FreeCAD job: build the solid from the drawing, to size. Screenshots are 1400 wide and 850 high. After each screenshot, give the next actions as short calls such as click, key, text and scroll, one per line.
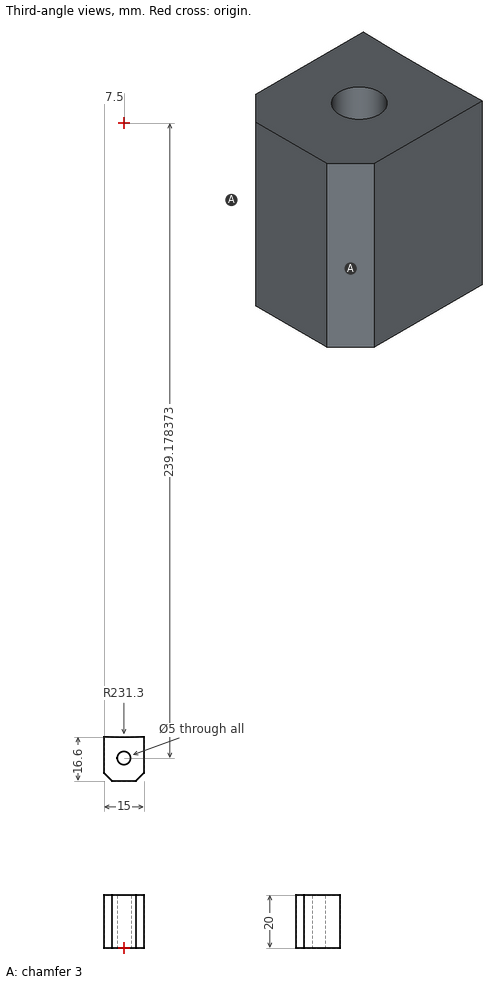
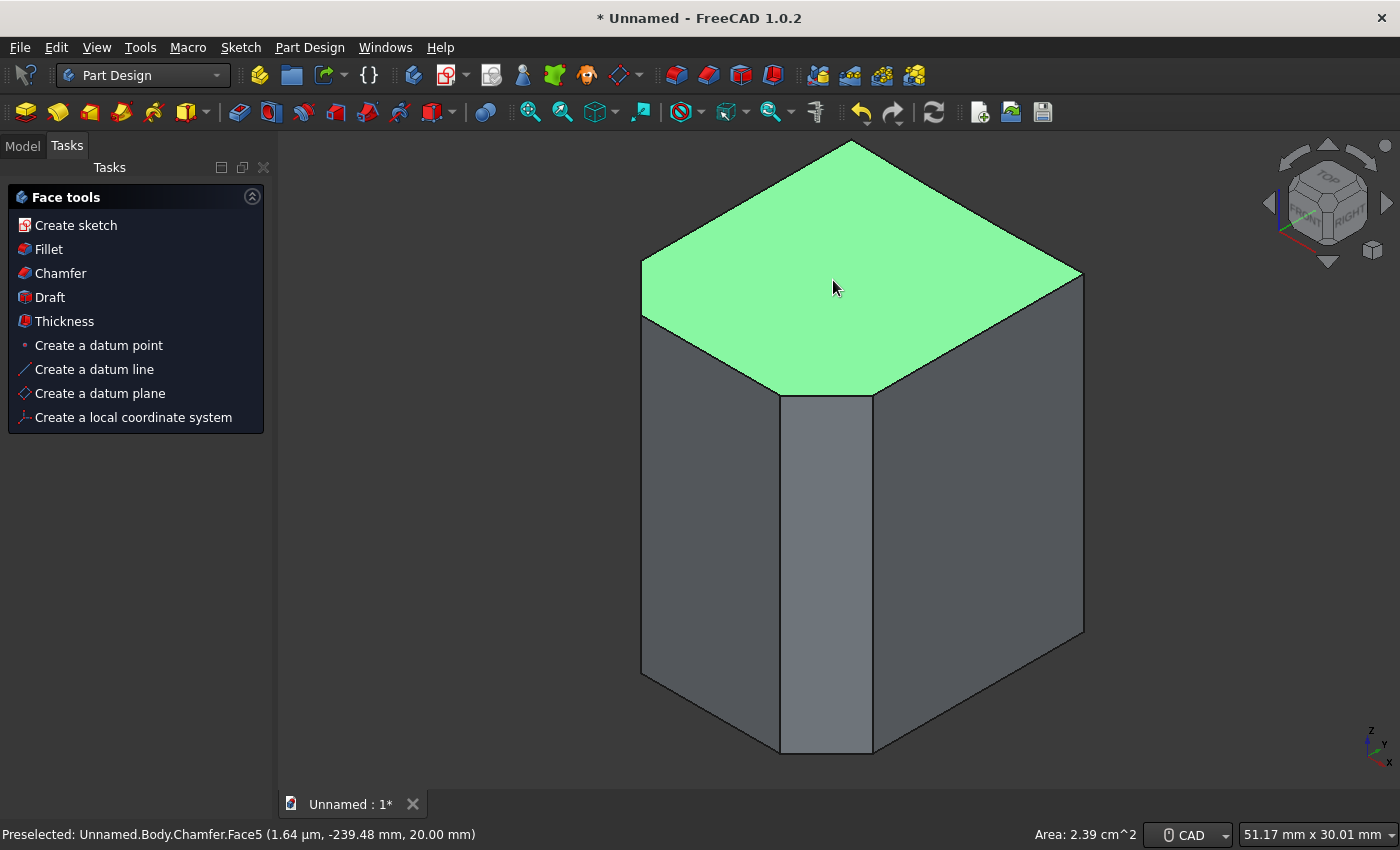
click(446, 76)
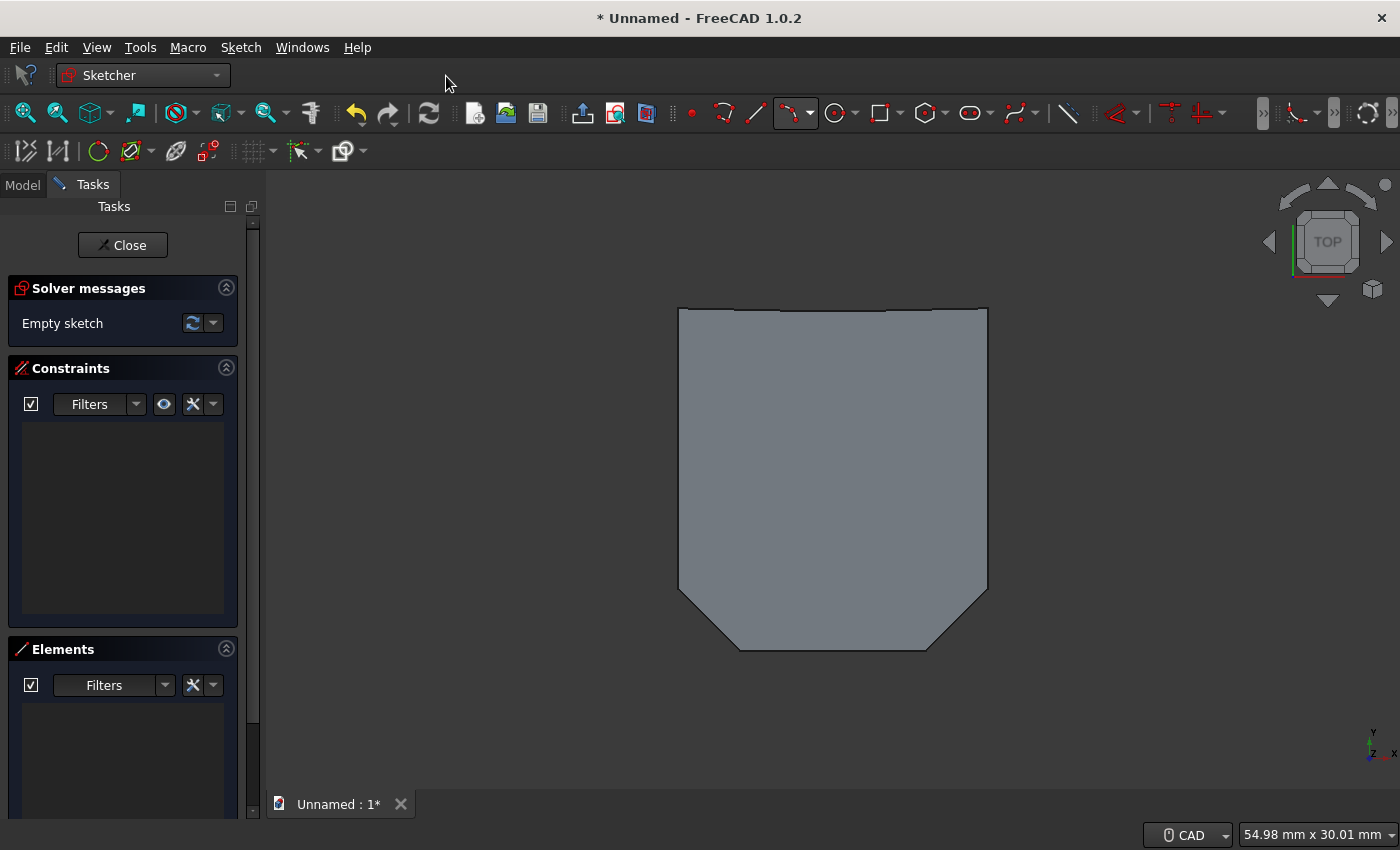
scroll(855, 471, up, 7)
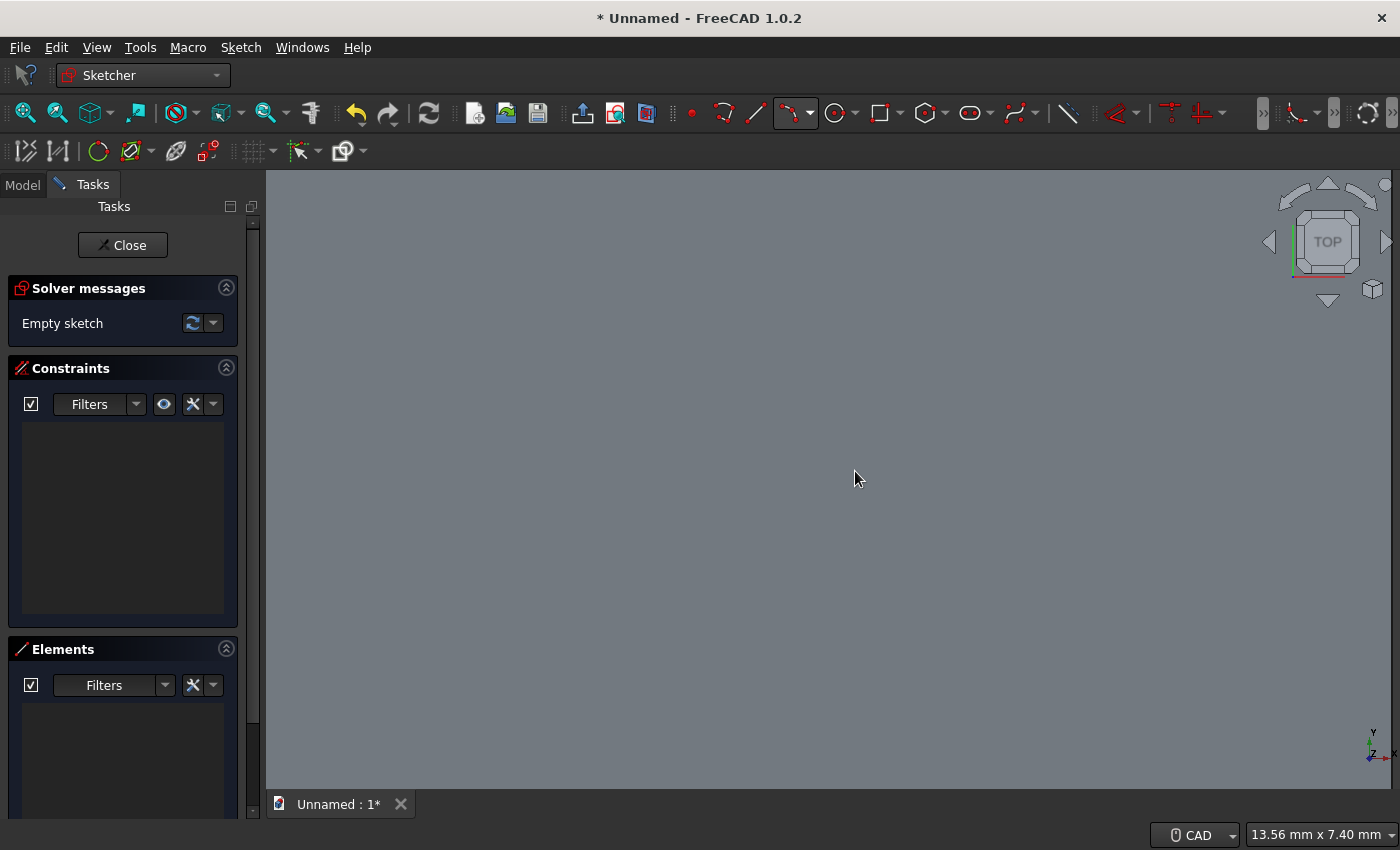
click(836, 114)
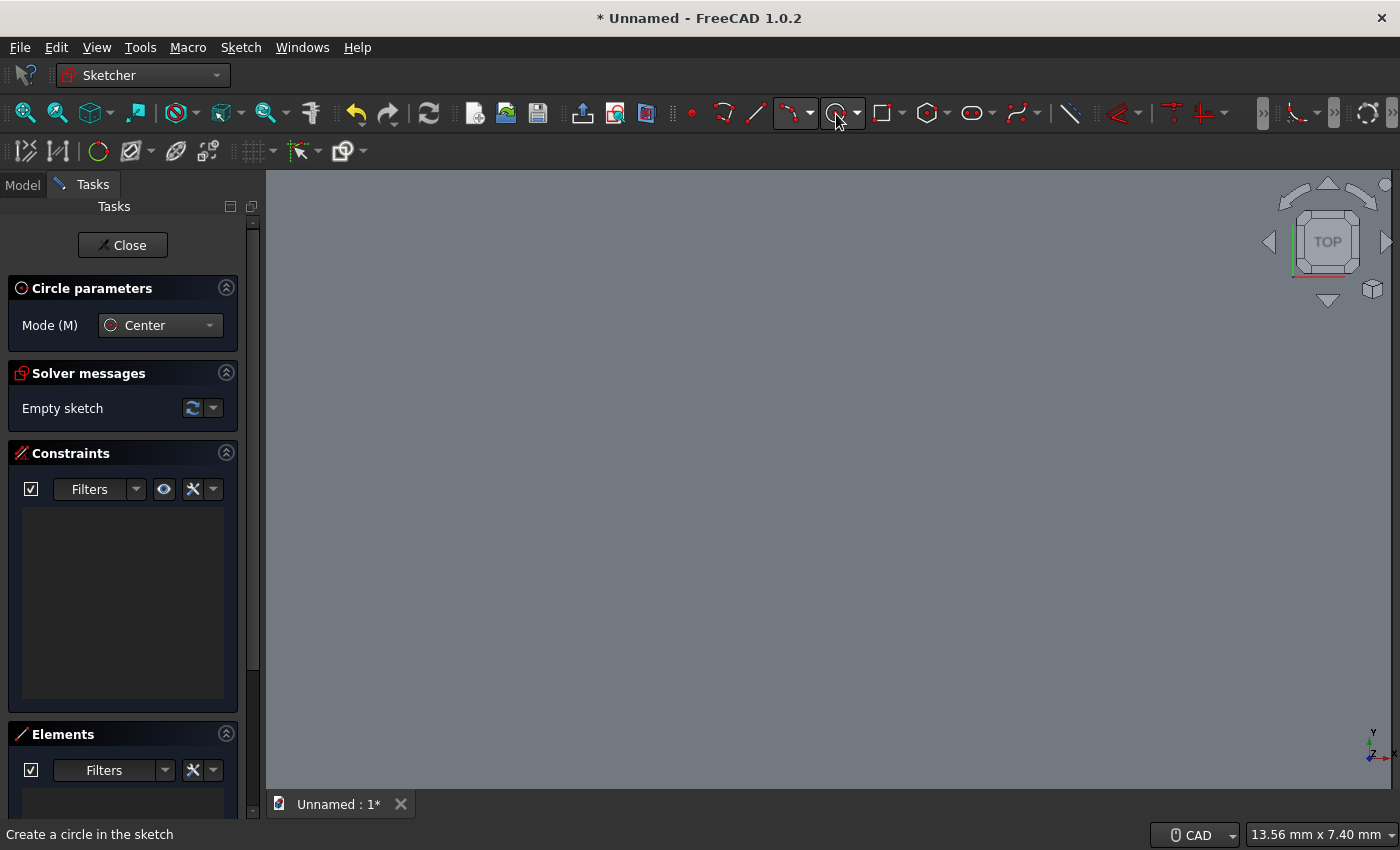
click(764, 479)
click(912, 331)
key(Escape)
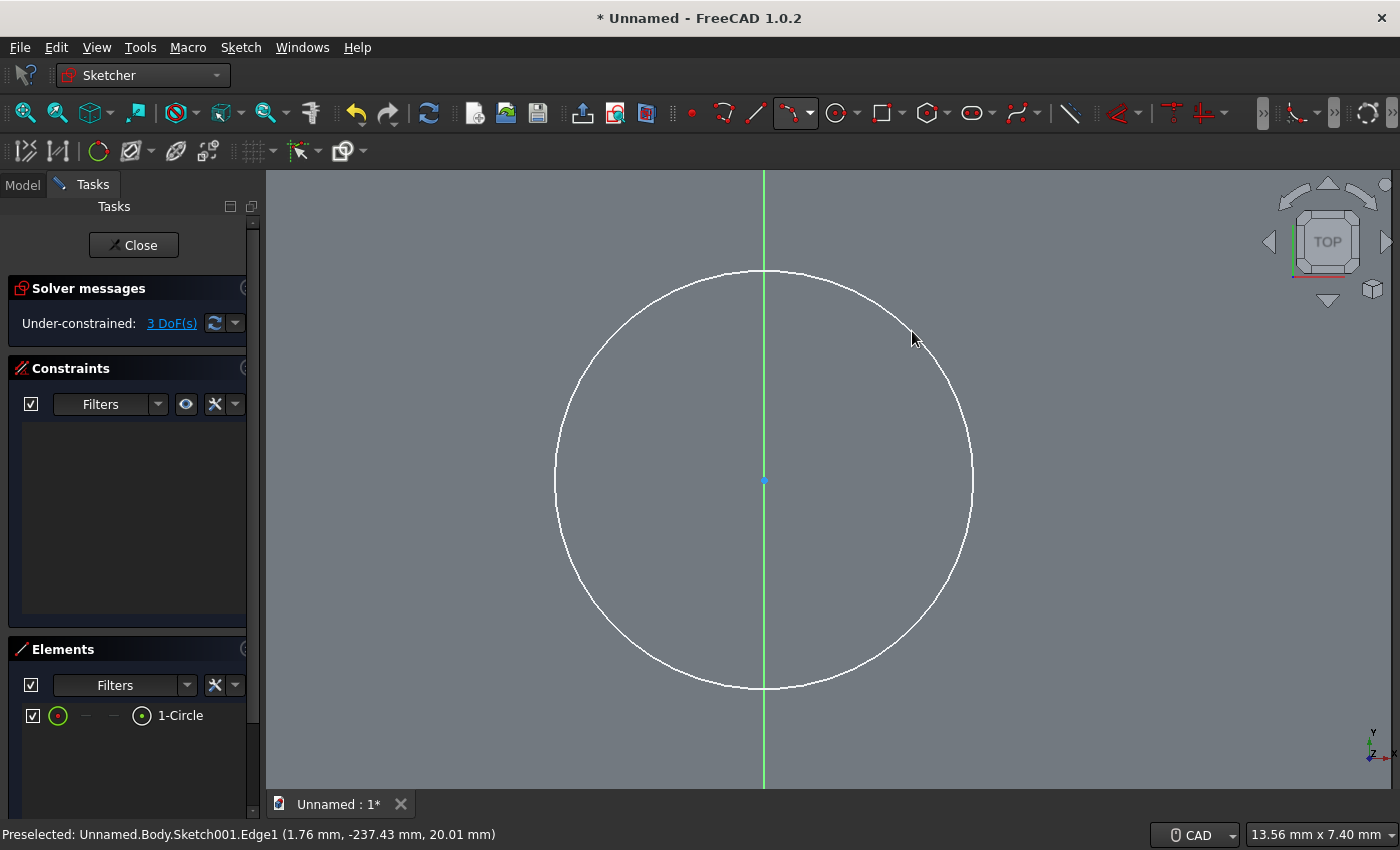
click(764, 480)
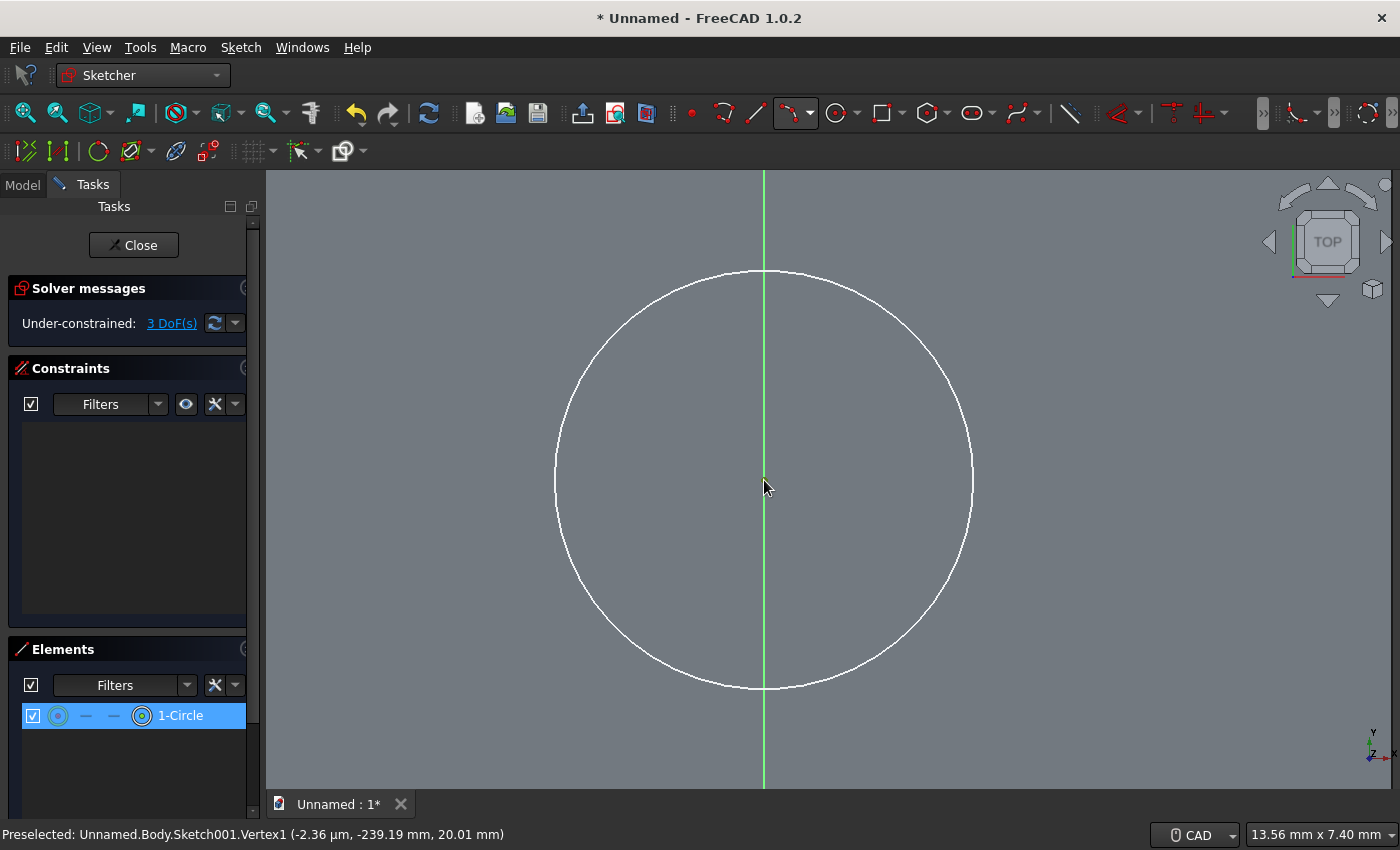
click(764, 721)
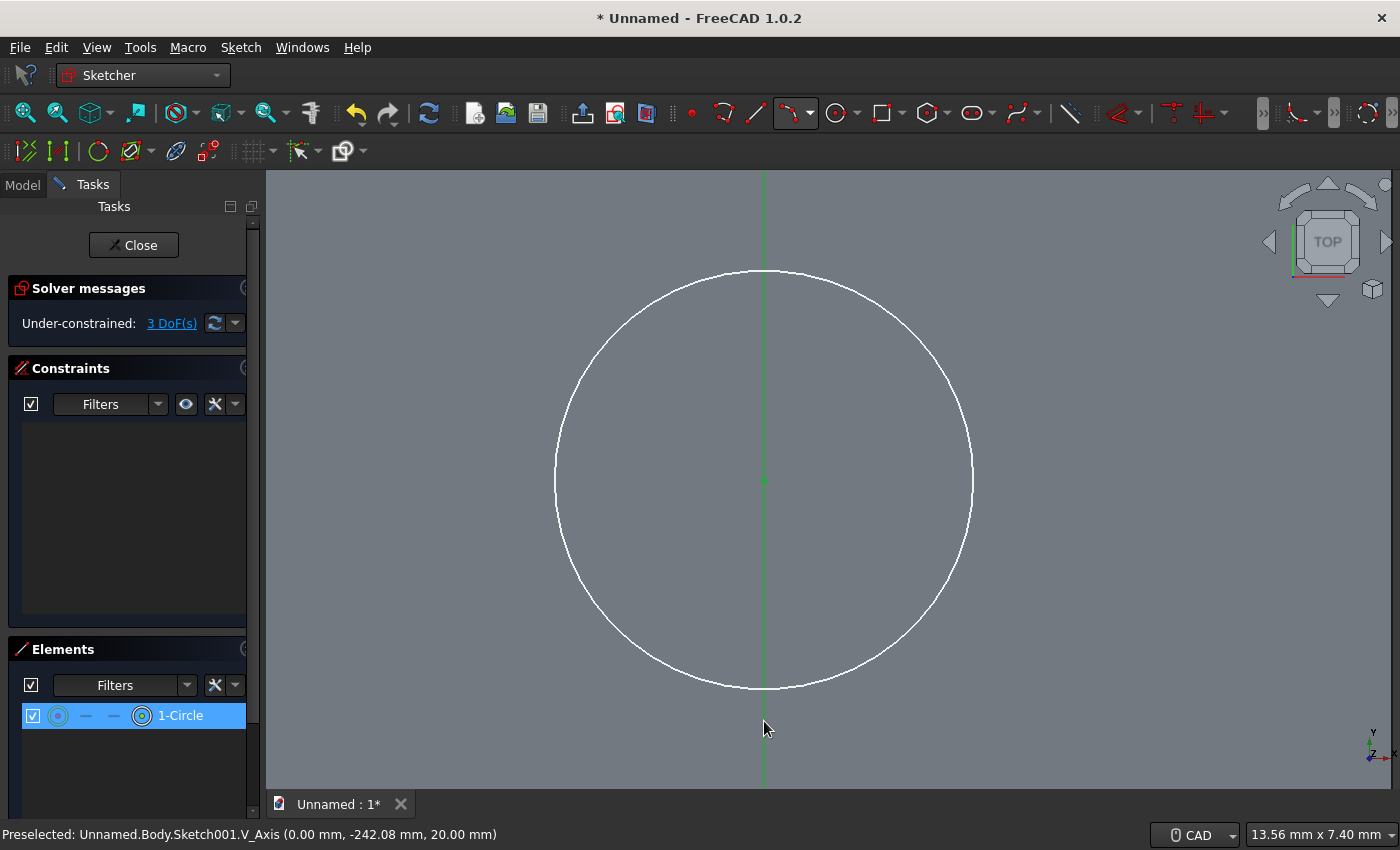
click(1172, 114)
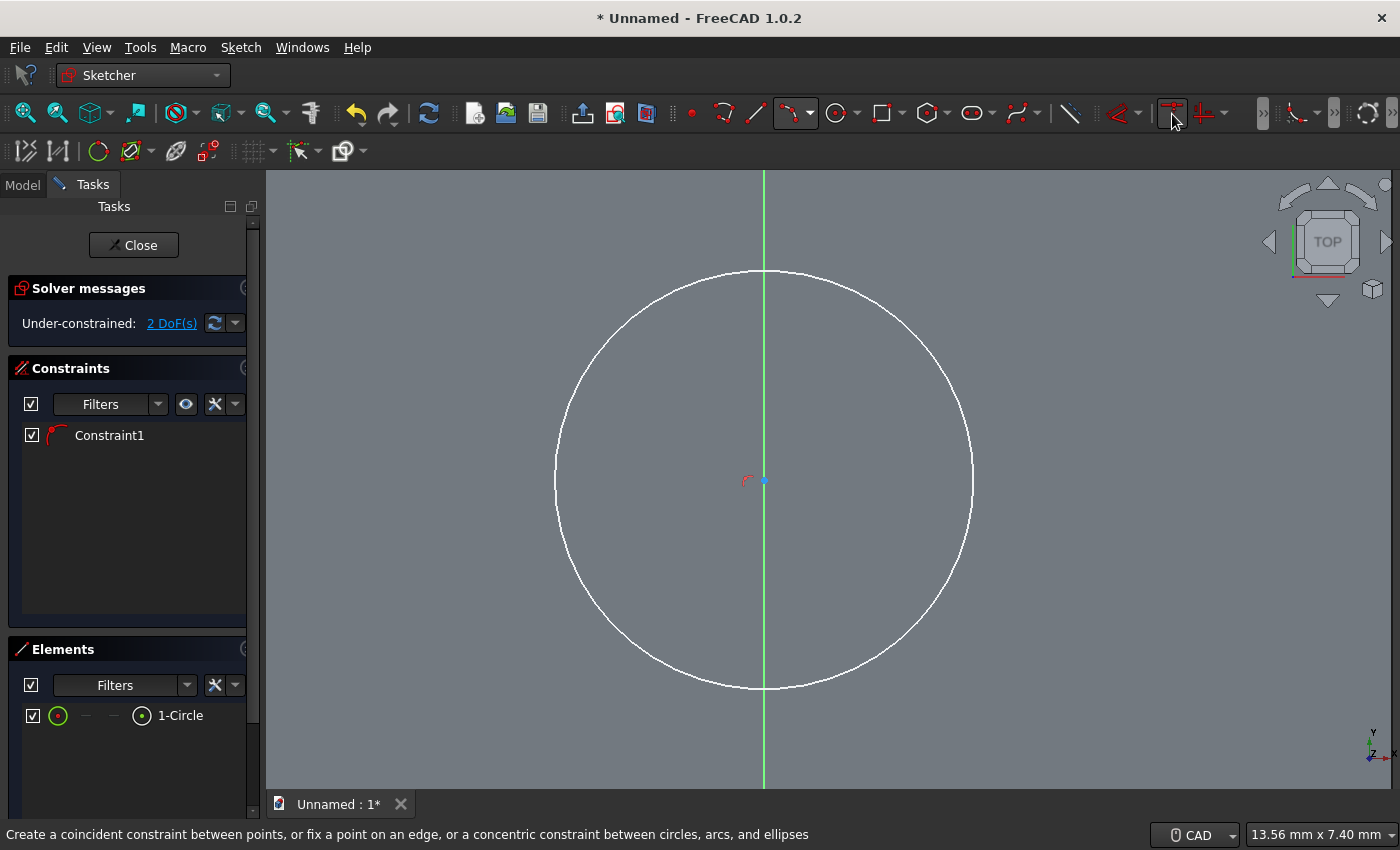
click(1118, 114)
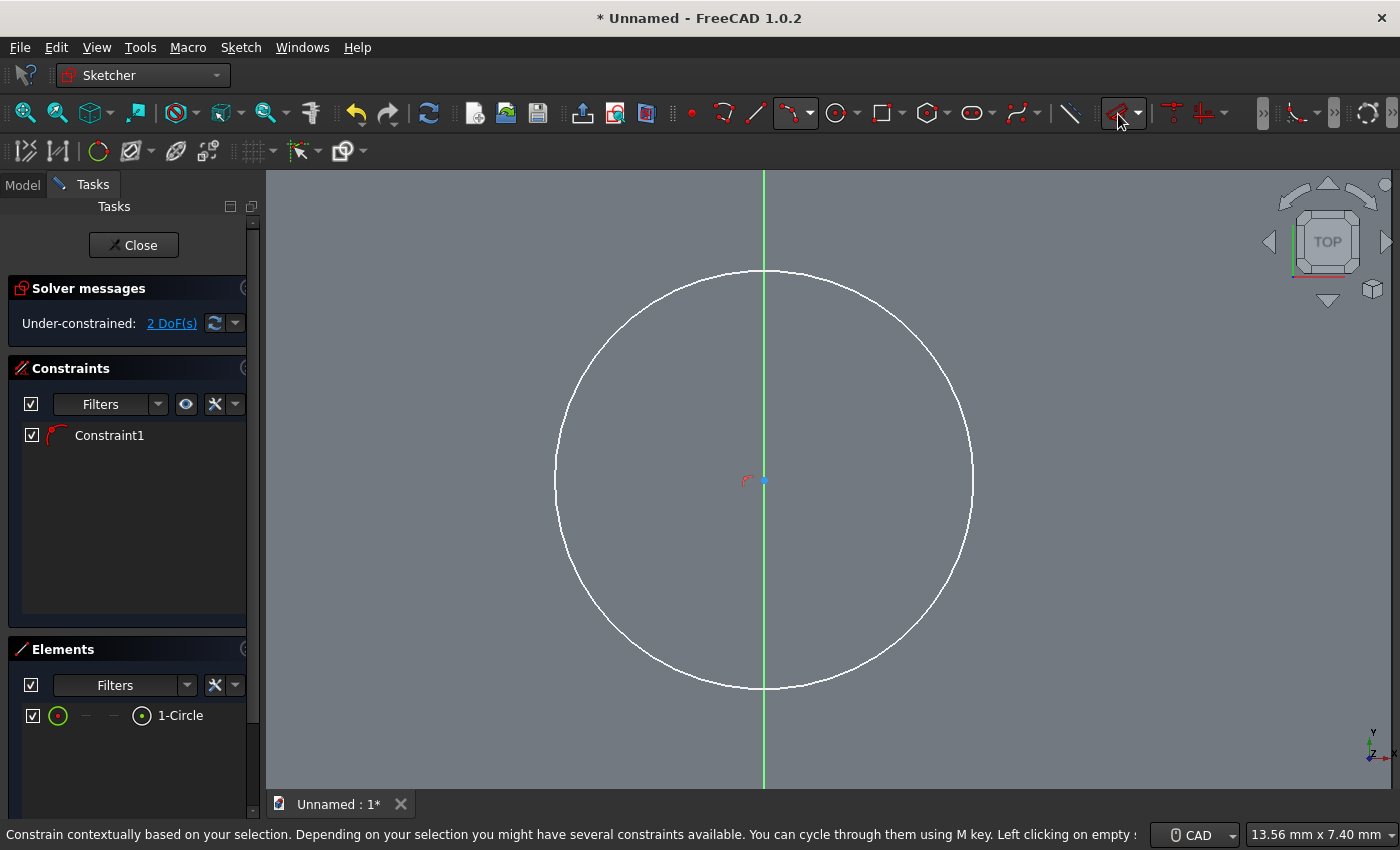
click(912, 332)
click(935, 309)